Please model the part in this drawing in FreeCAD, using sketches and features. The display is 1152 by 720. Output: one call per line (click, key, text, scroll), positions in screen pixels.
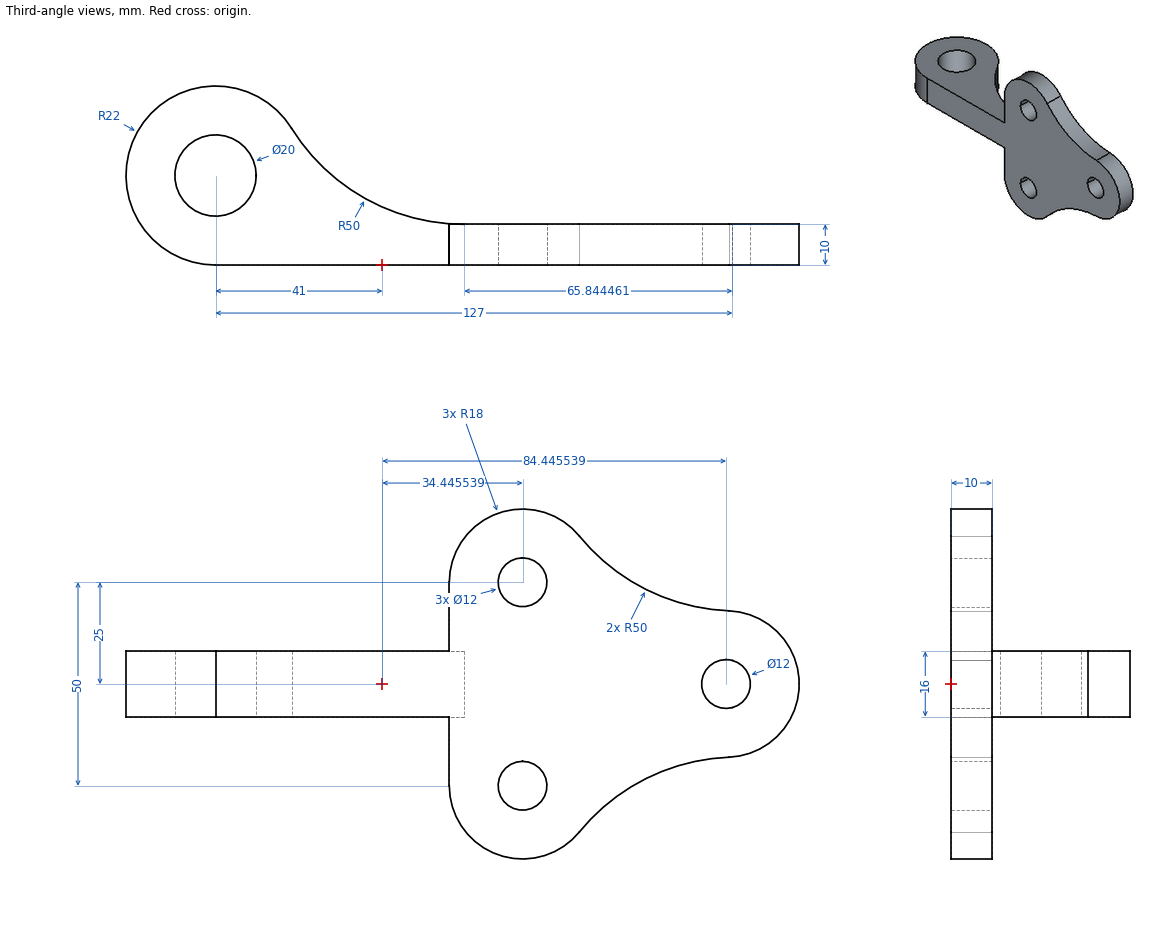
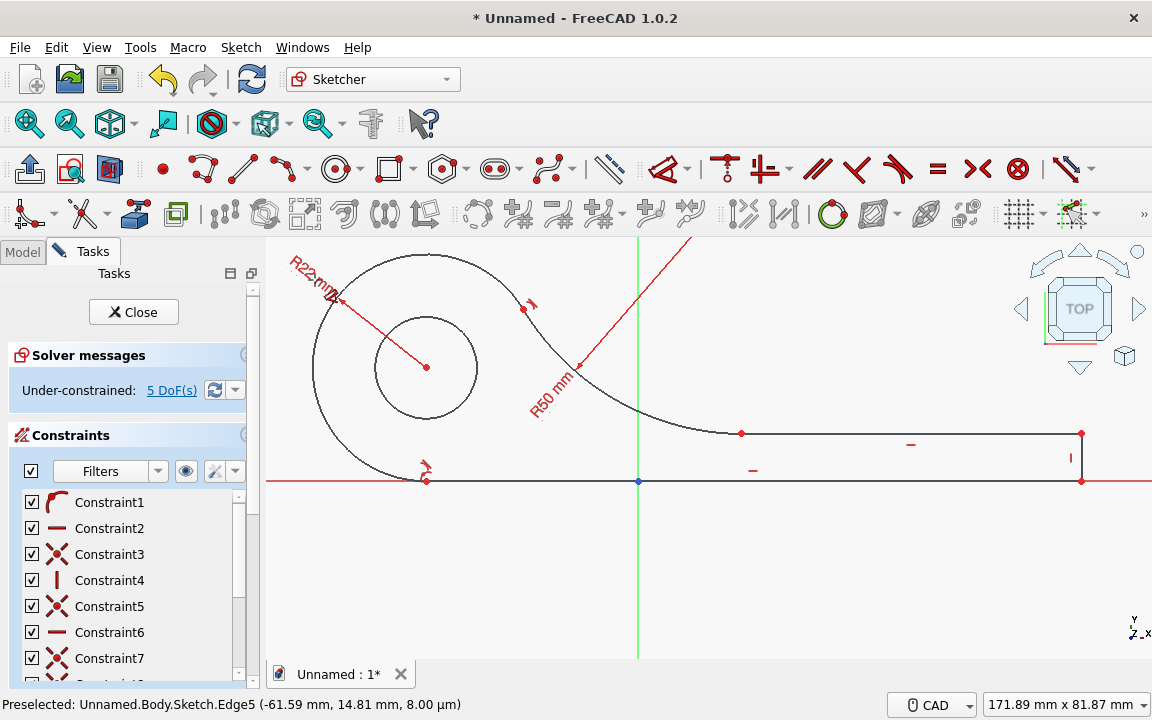
click(462, 332)
click(485, 309)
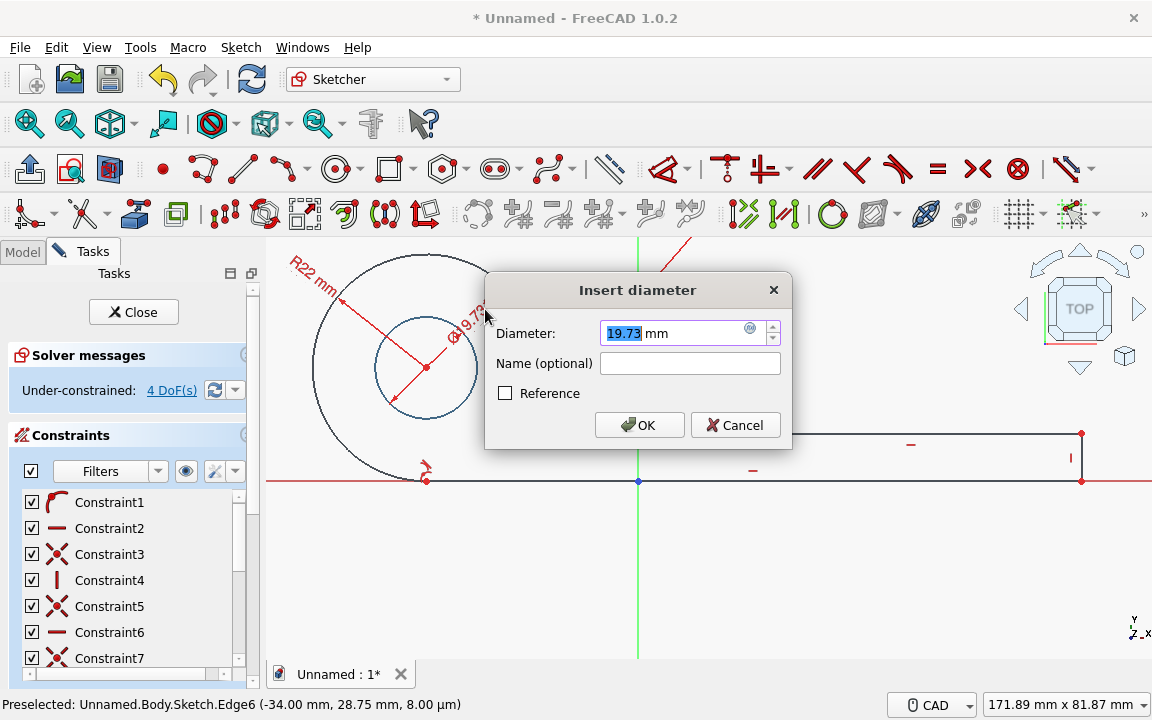
text(20)
key(Return)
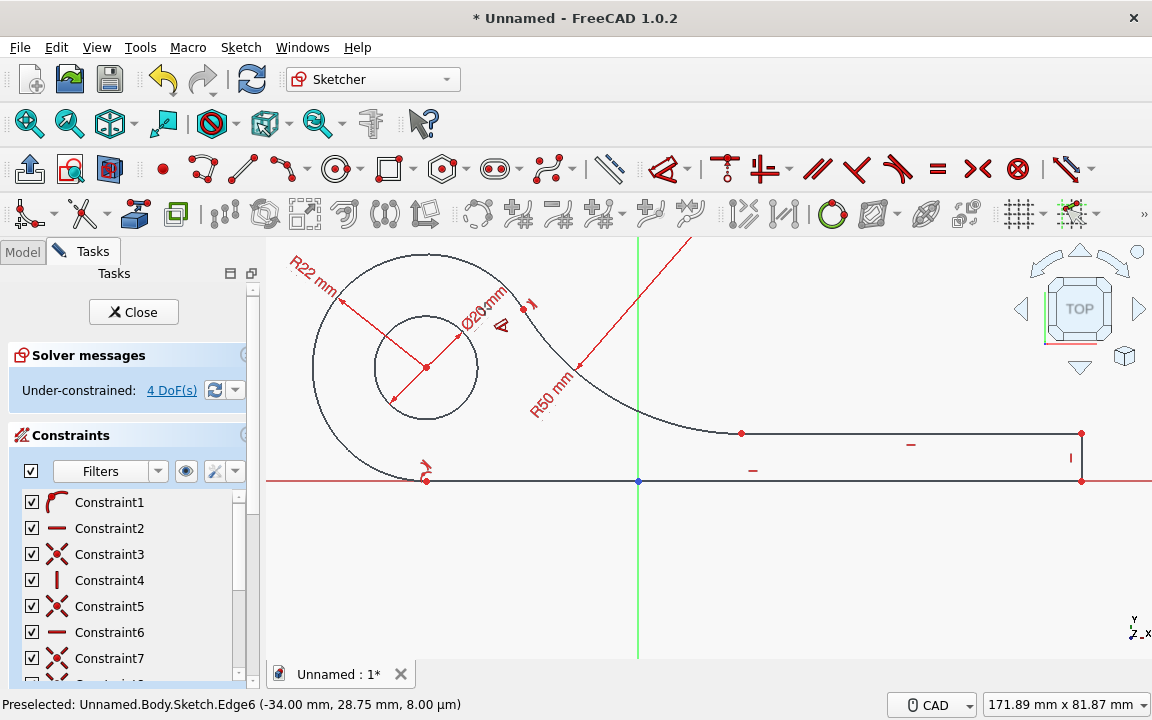
scroll(510, 557, down, 2)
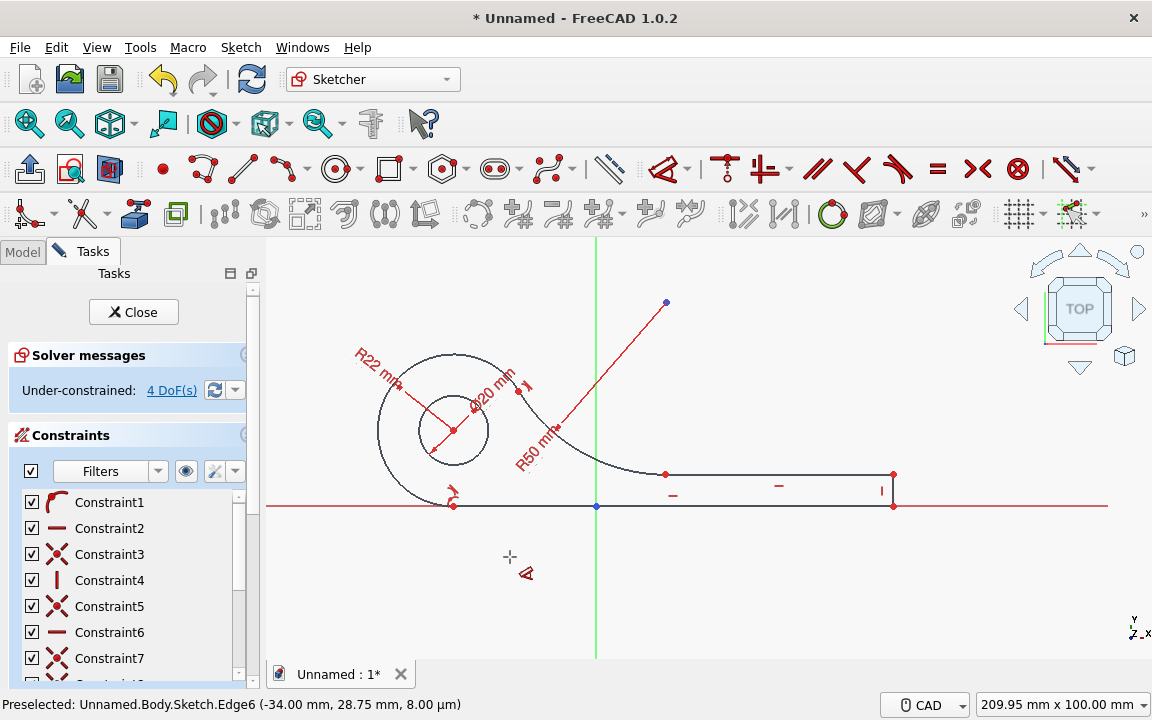
scroll(893, 497, up, 2)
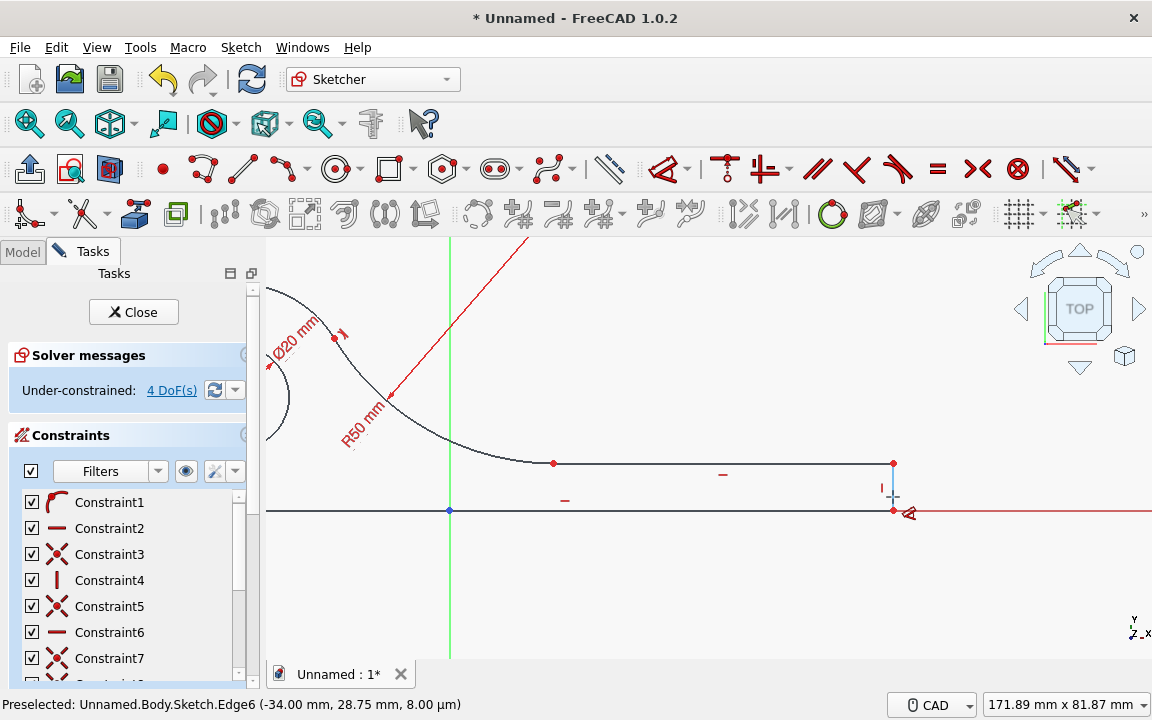
click(893, 497)
click(927, 487)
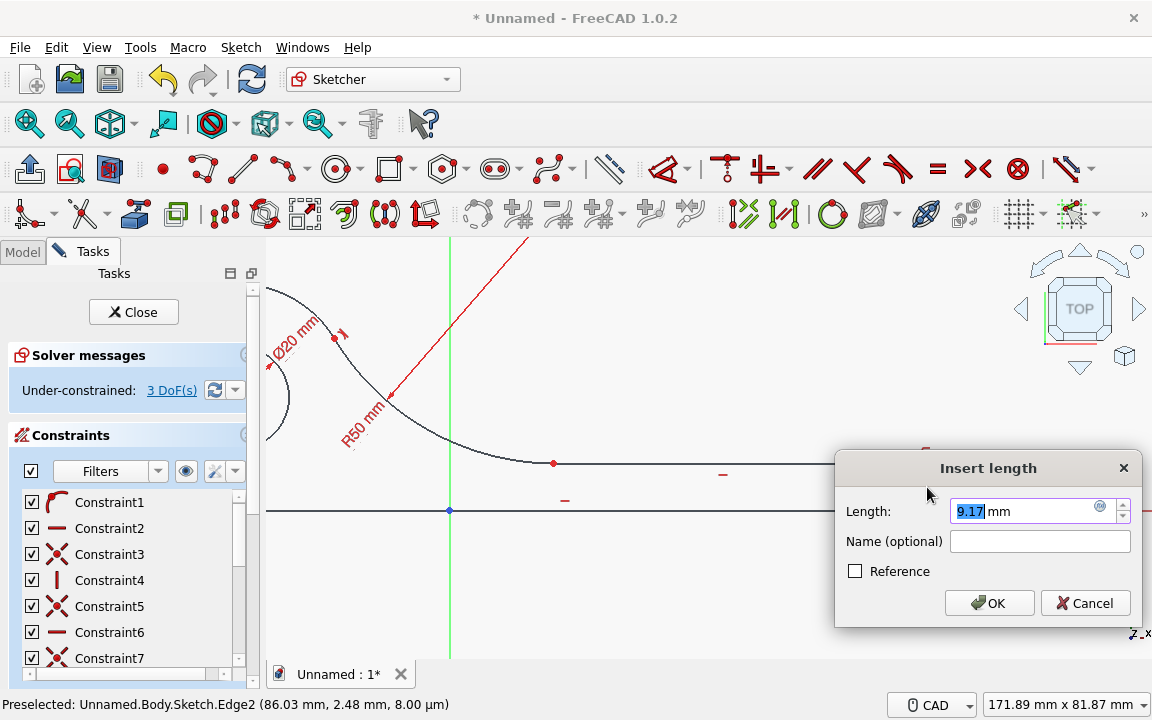
text(10)
key(Return)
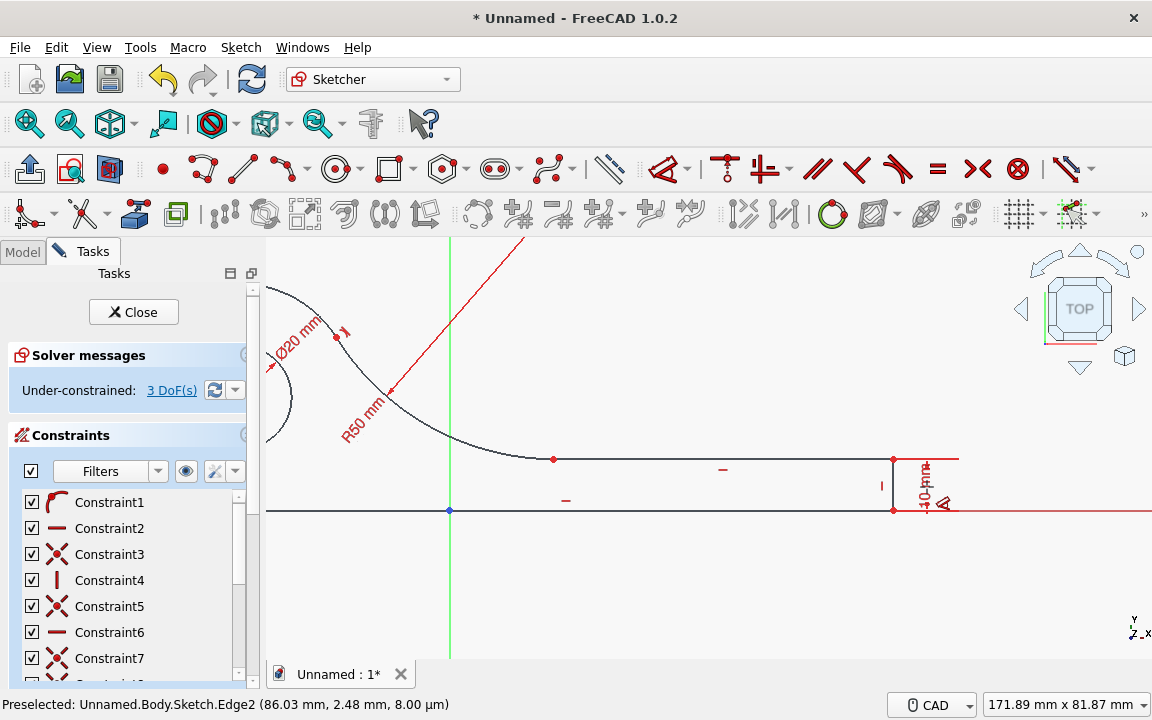
scroll(893, 496, down, 2)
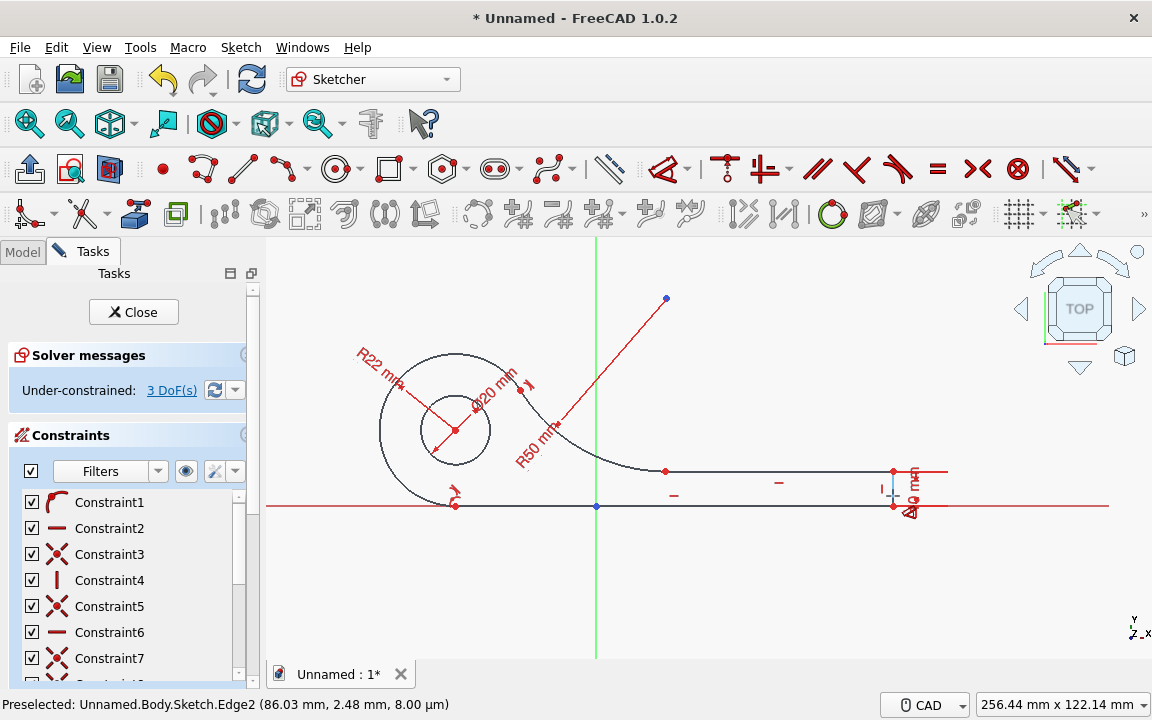
click(456, 430)
click(526, 540)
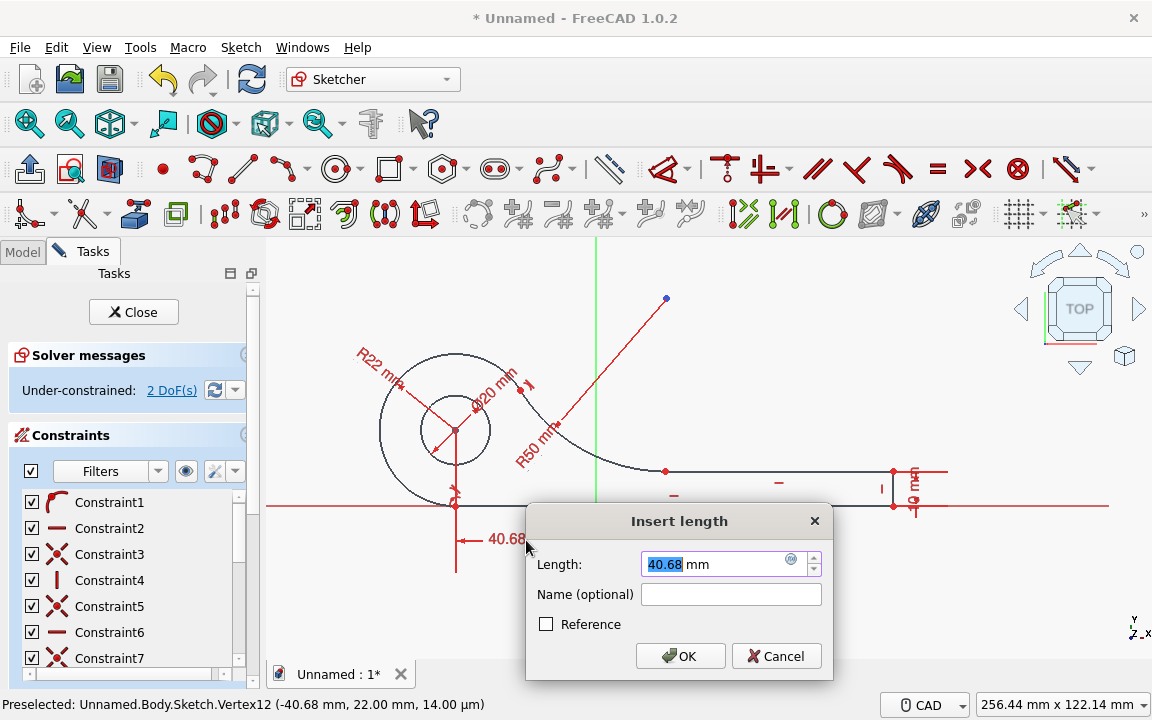
text(41)
key(Return)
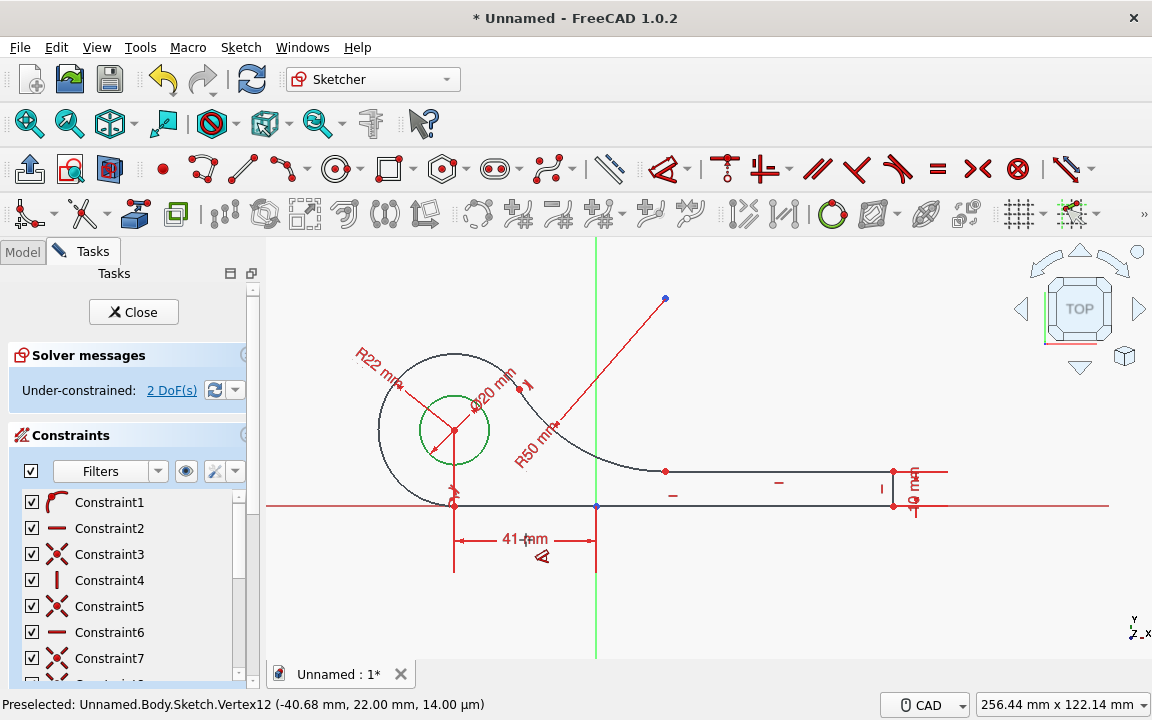
scroll(586, 506, up, 2)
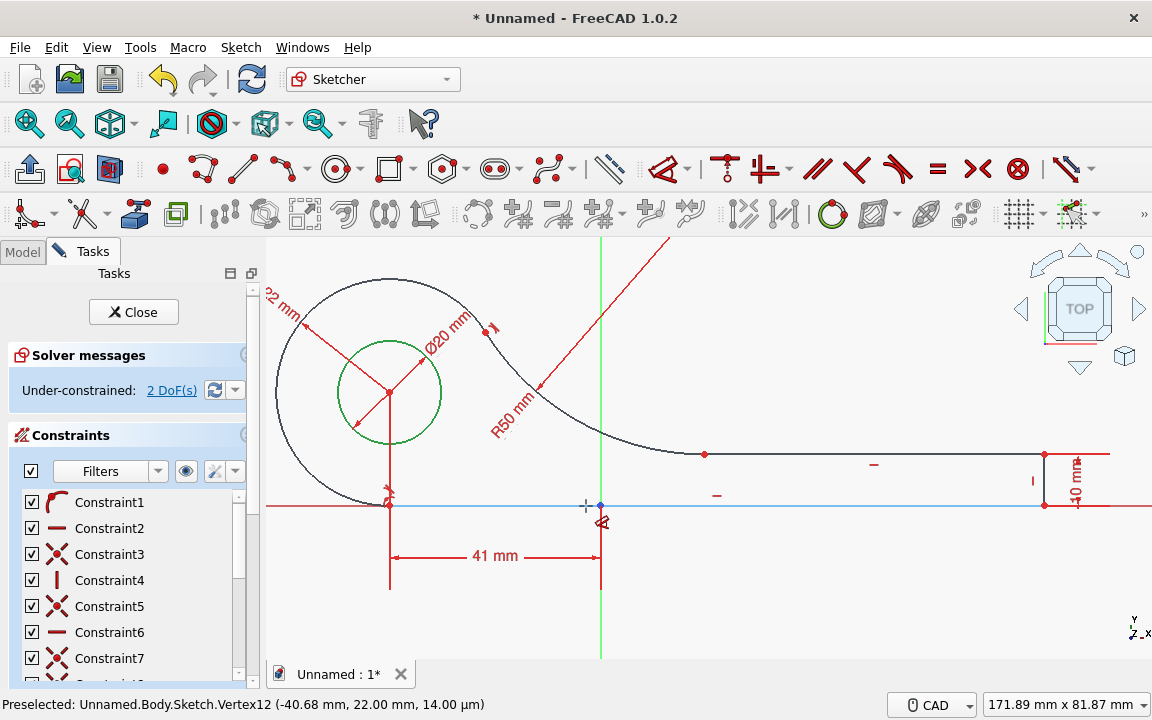
click(586, 506)
click(688, 540)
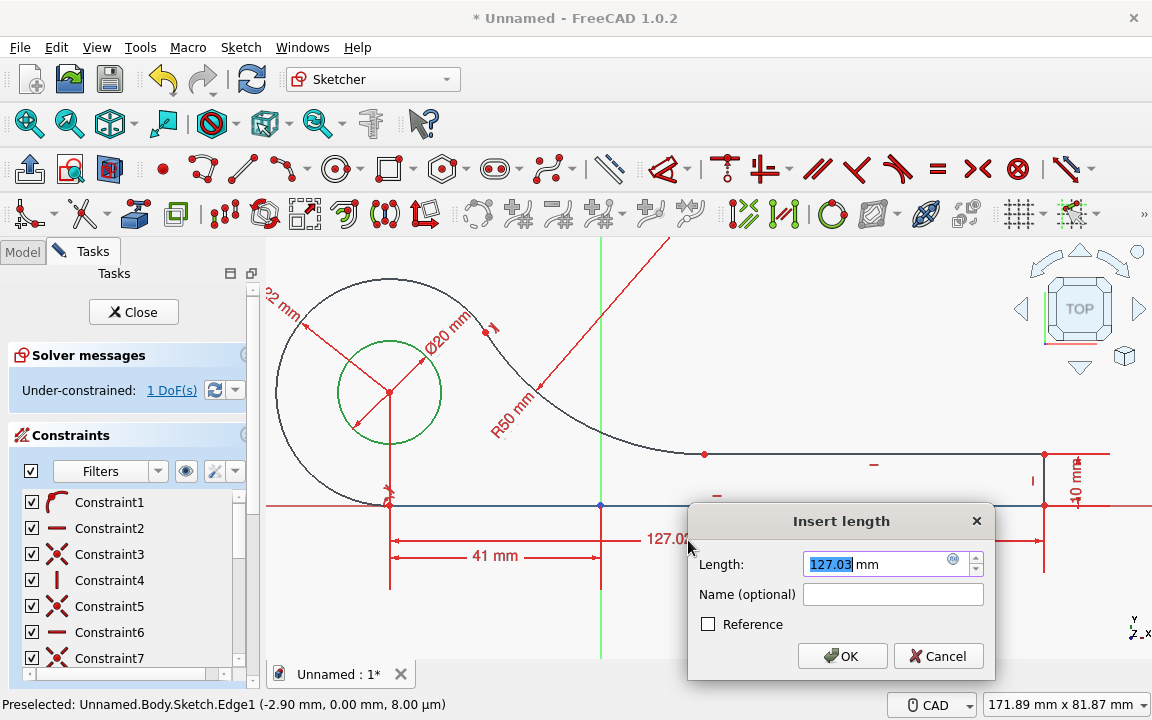
text(127)
key(Return)